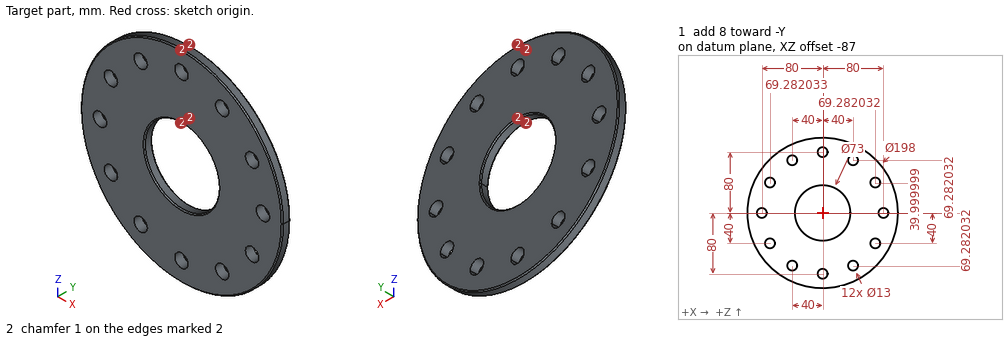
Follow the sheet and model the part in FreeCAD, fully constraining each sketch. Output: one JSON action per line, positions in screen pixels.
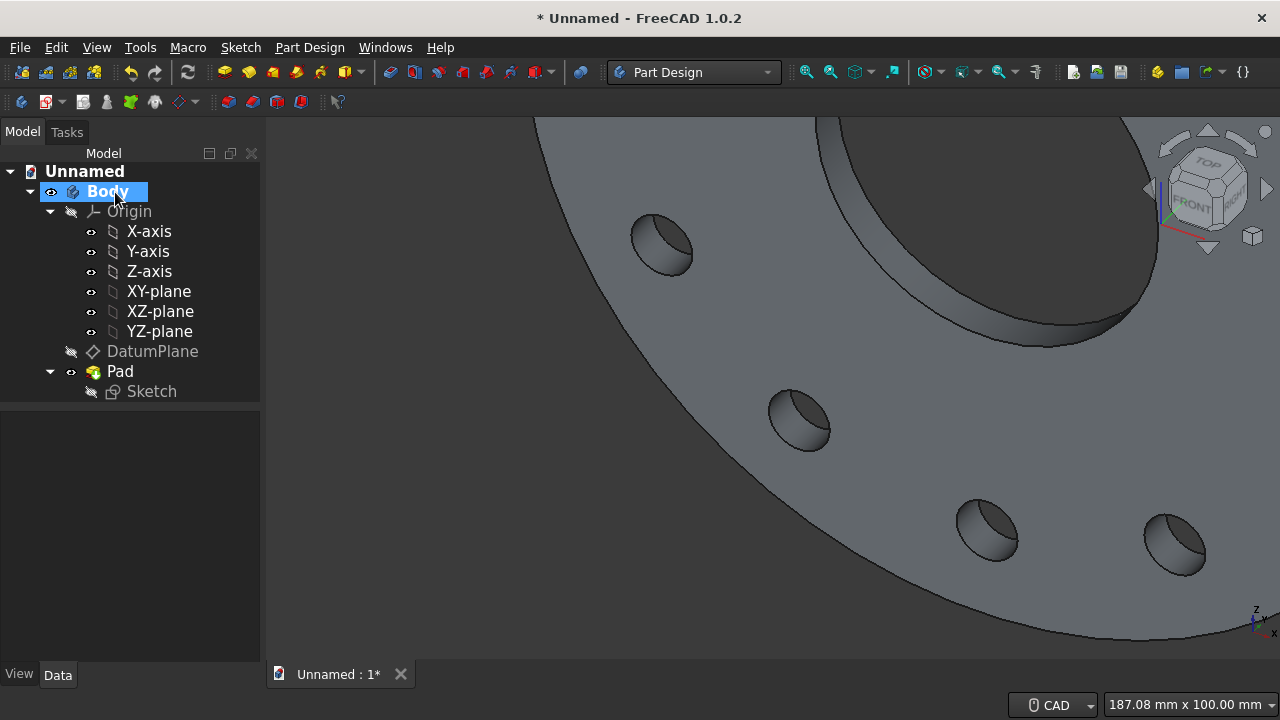
{"action": "key", "text": "v f"}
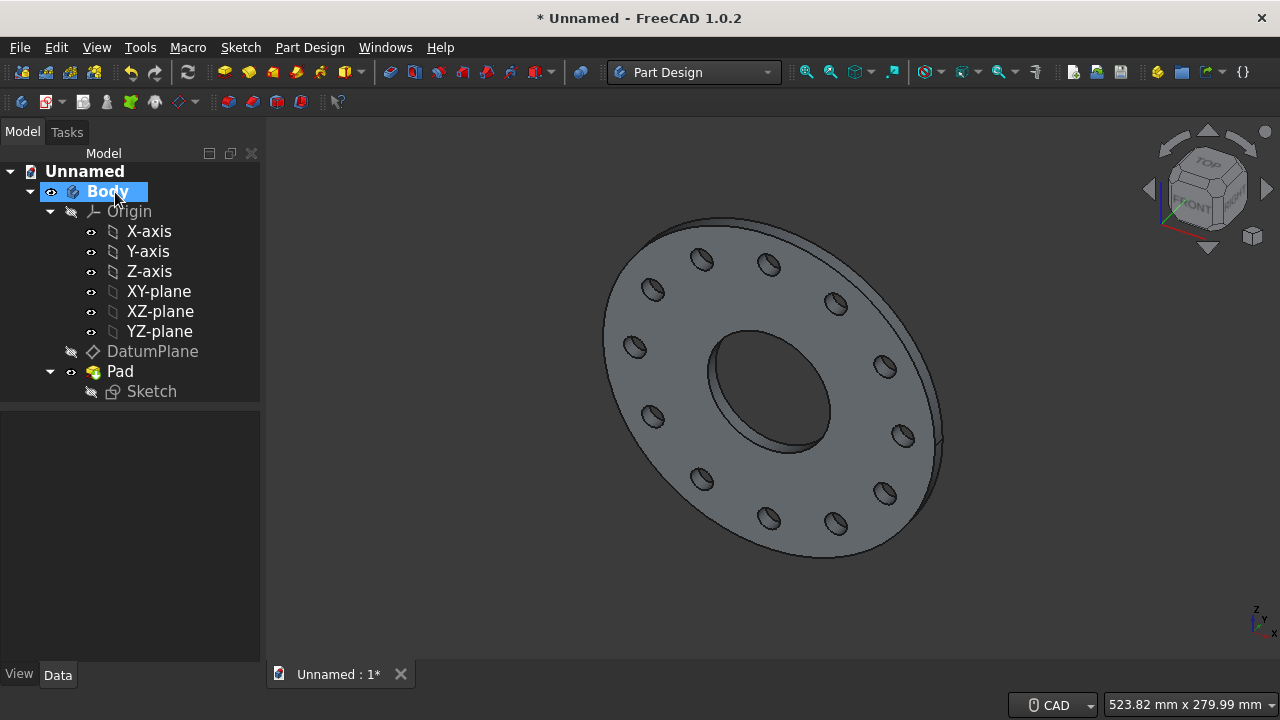
{"action": "left_click", "coordinate": [940, 408]}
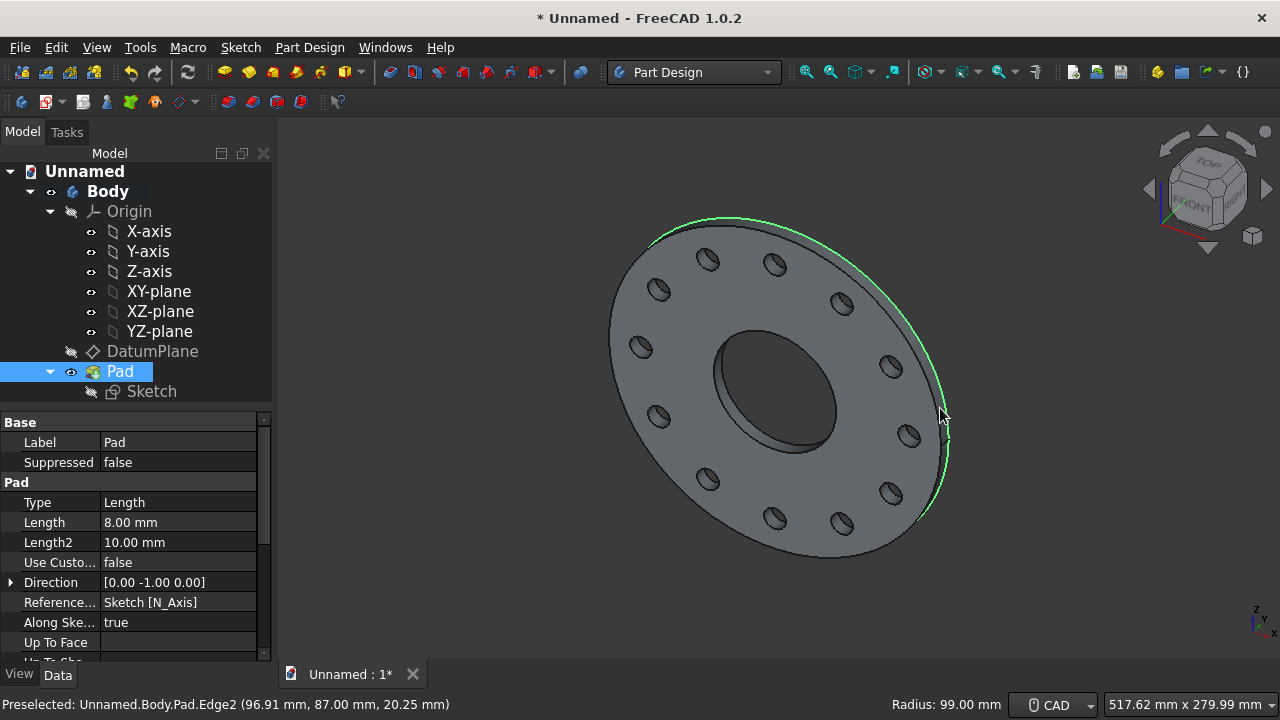
{"action": "left_click", "coordinate": [724, 225], "text": "ctrl"}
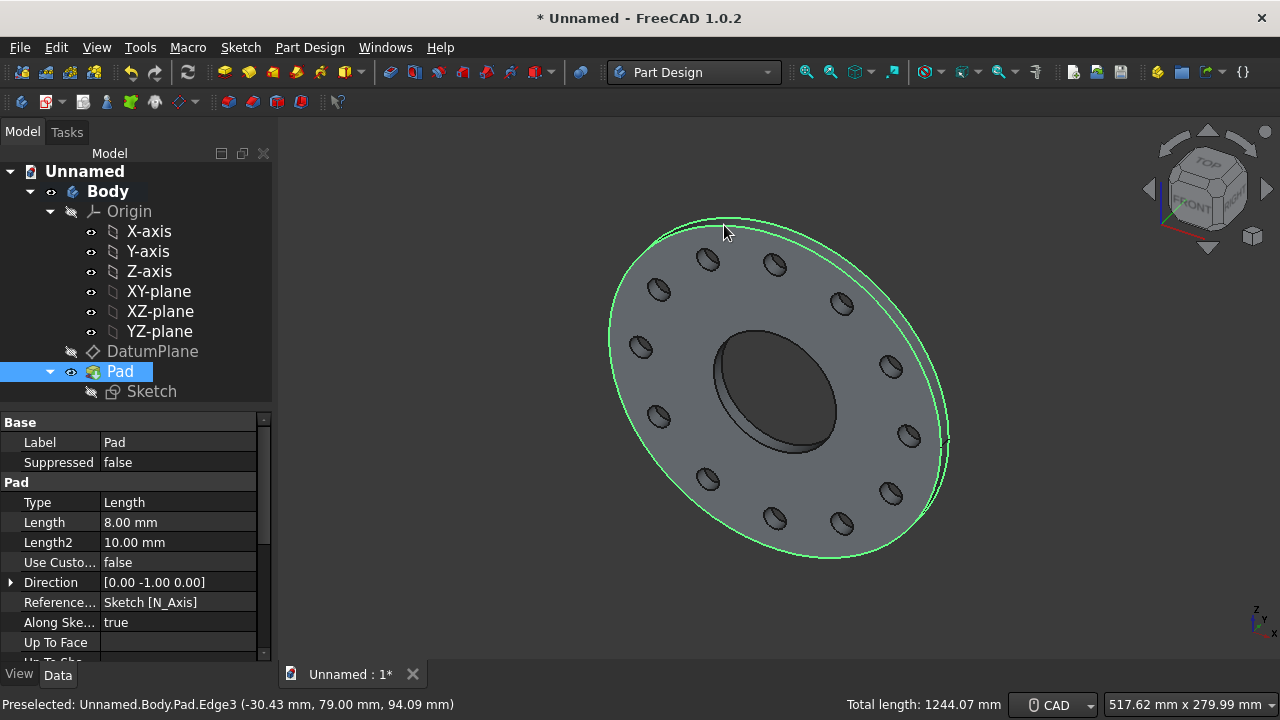
{"action": "left_click", "coordinate": [714, 371], "text": "ctrl"}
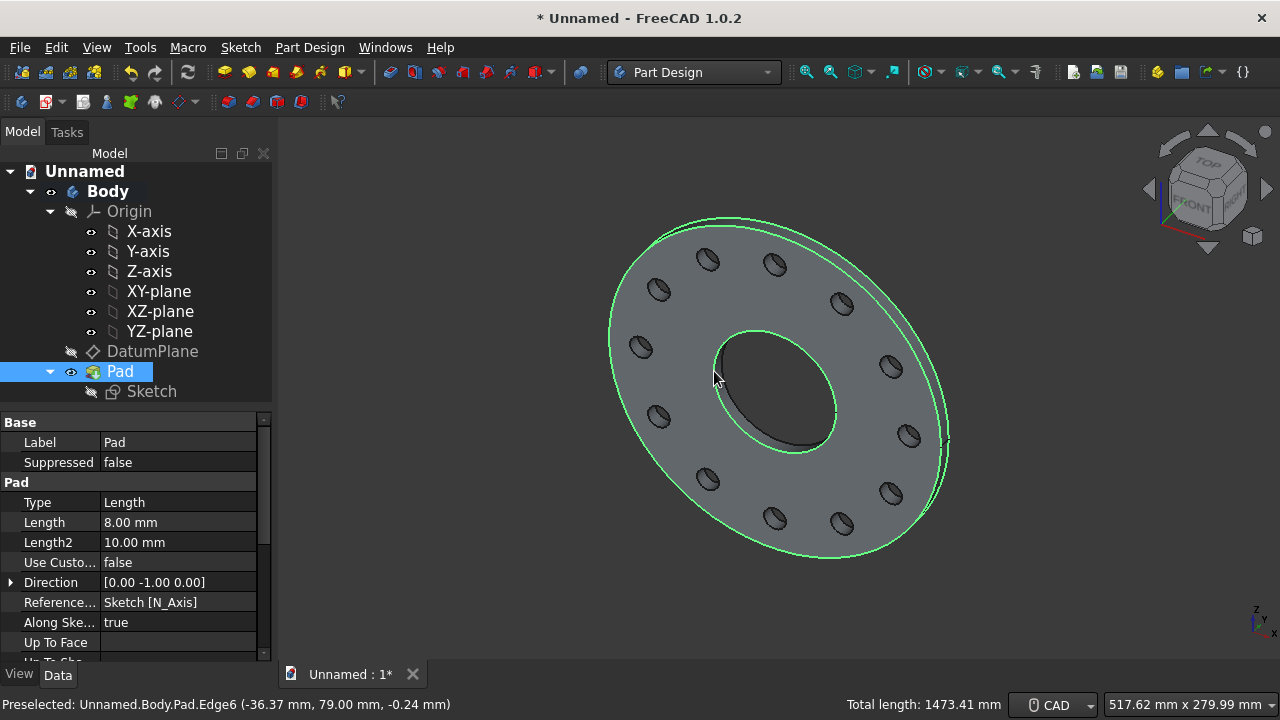
{"action": "key", "text": "0"}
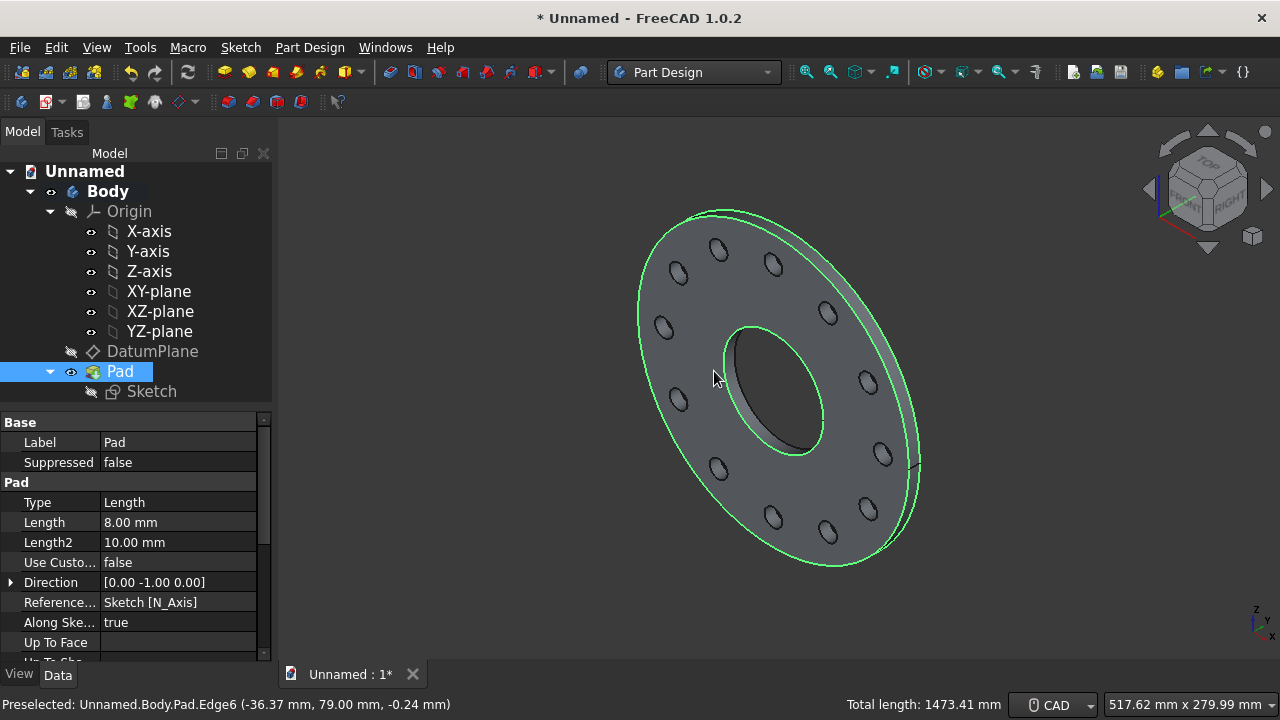
{"action": "key", "text": "2"}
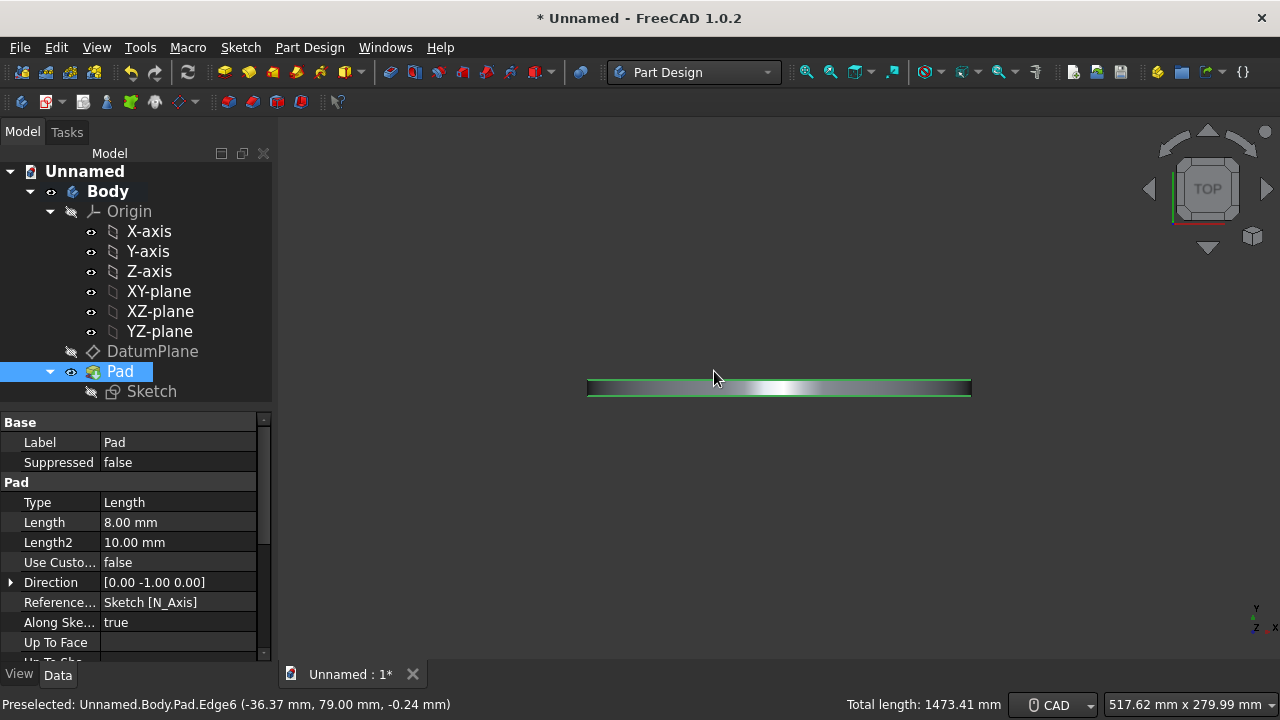
{"action": "left_click", "coordinate": [808, 72]}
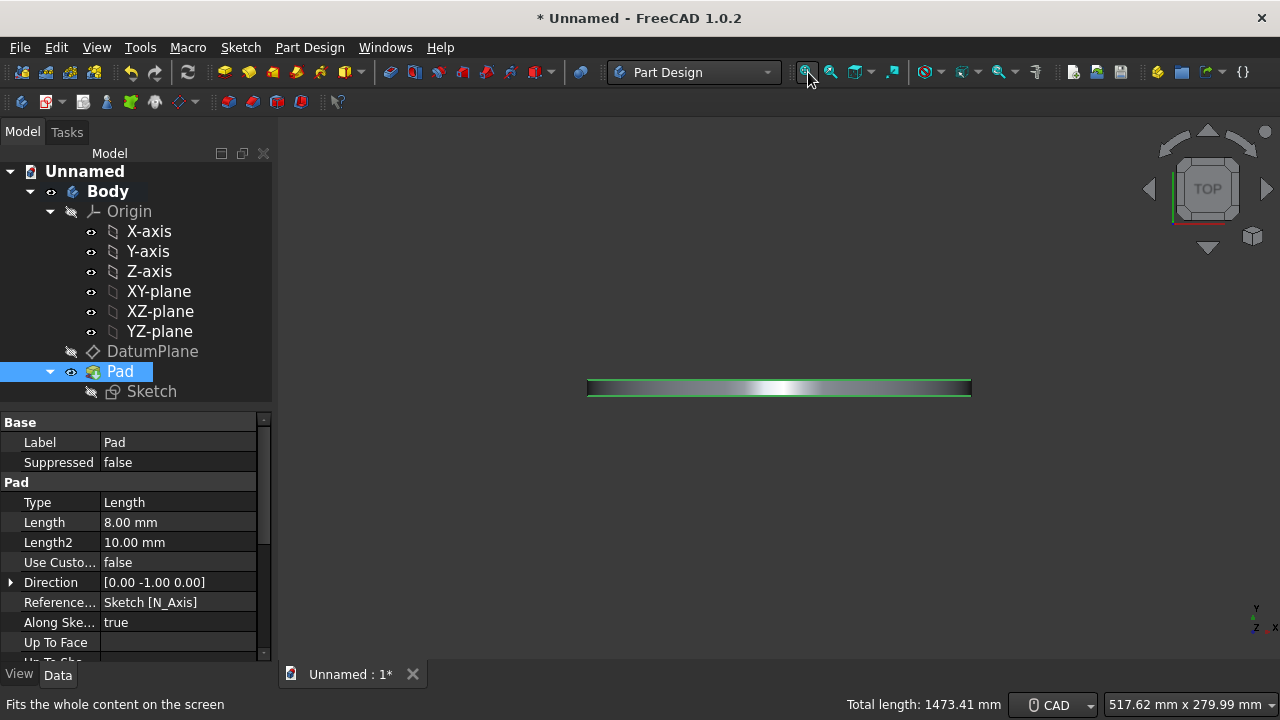
{"action": "key", "text": "1"}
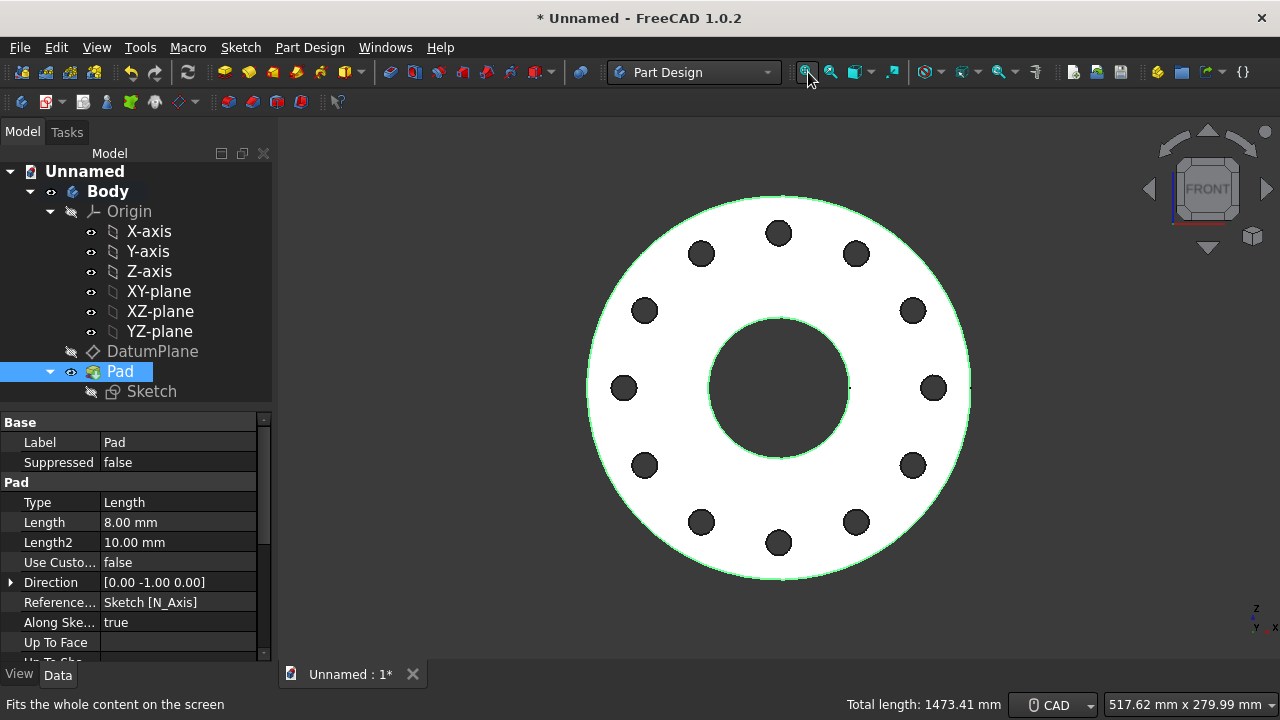
{"action": "key", "text": "3"}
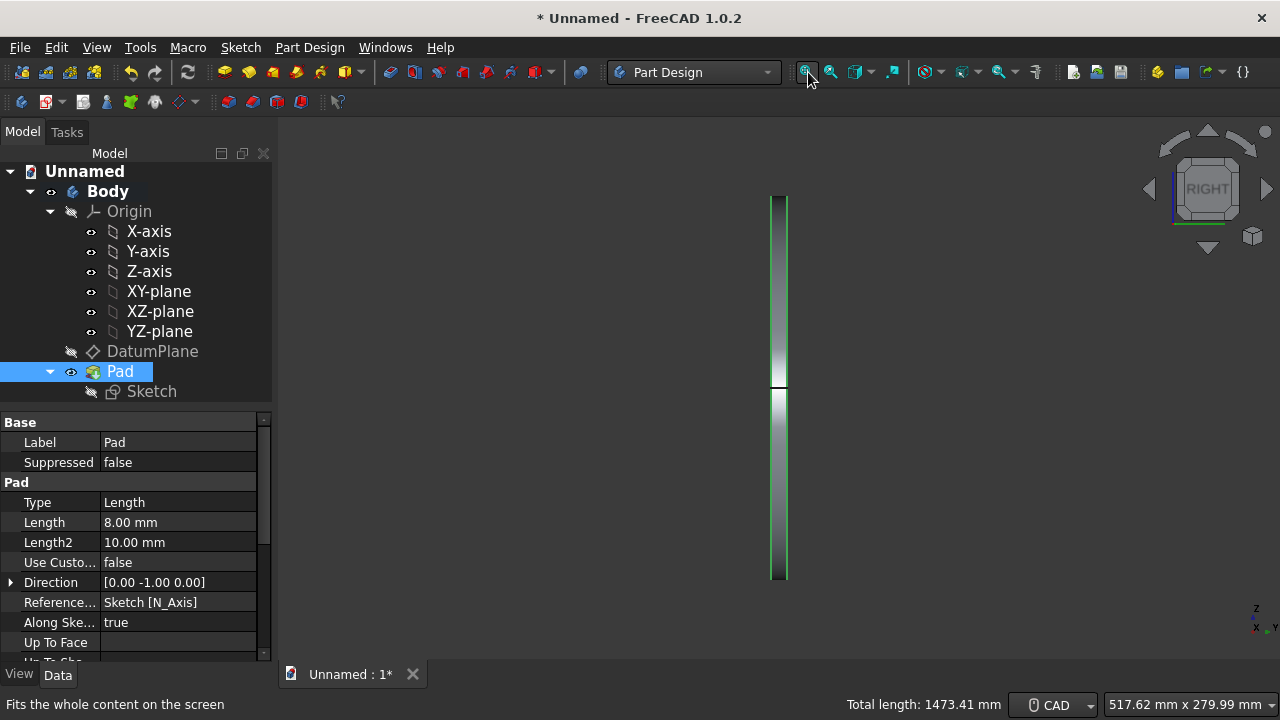
{"action": "key", "text": "5"}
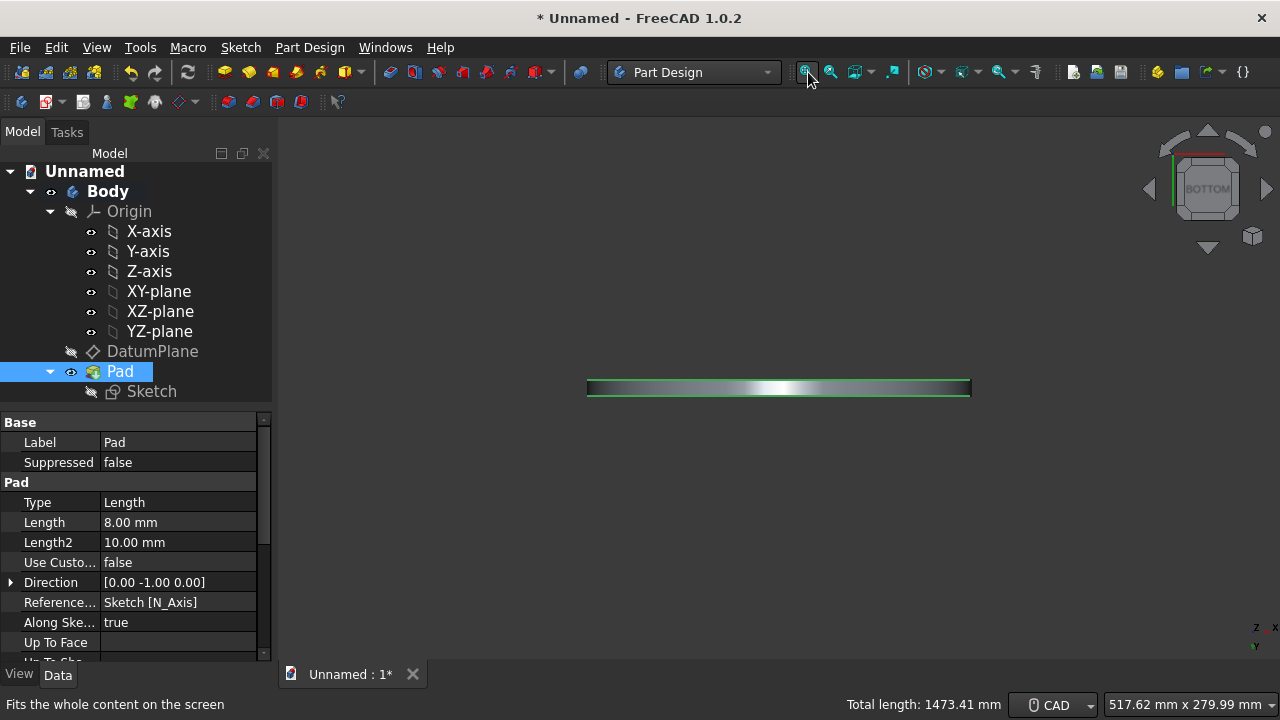
{"action": "key", "text": "v f"}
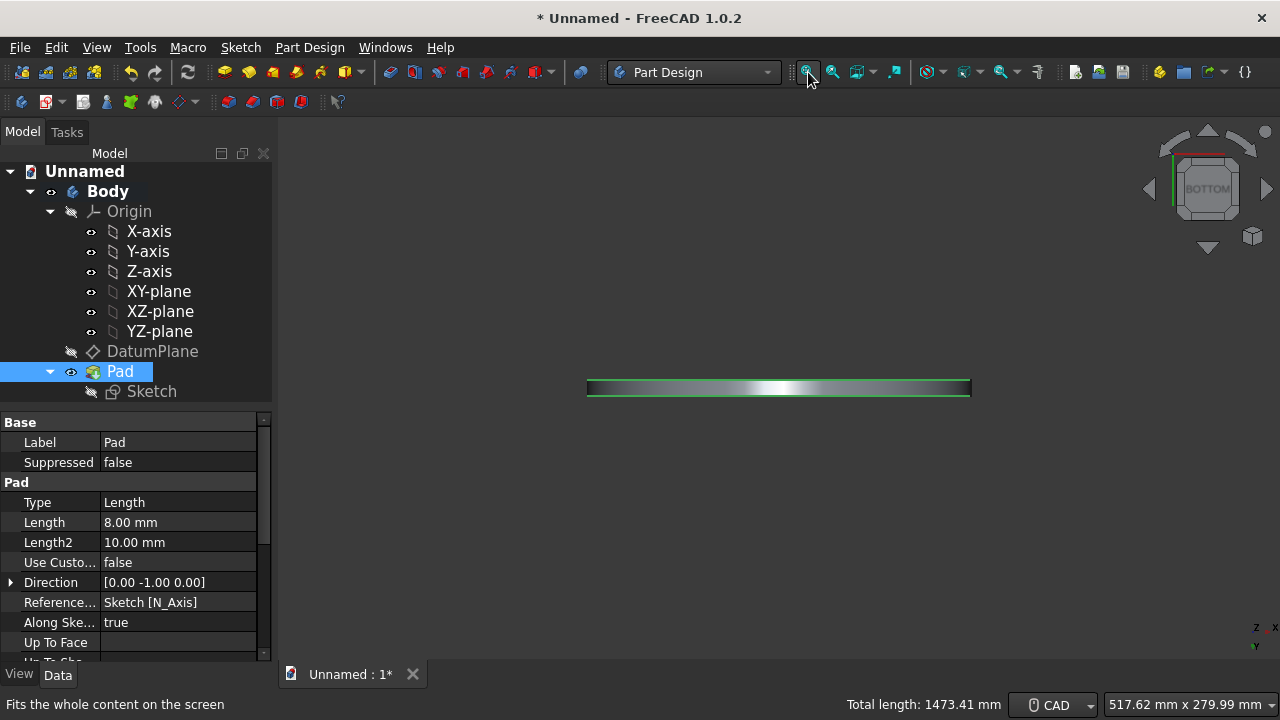
{"action": "key", "text": "4"}